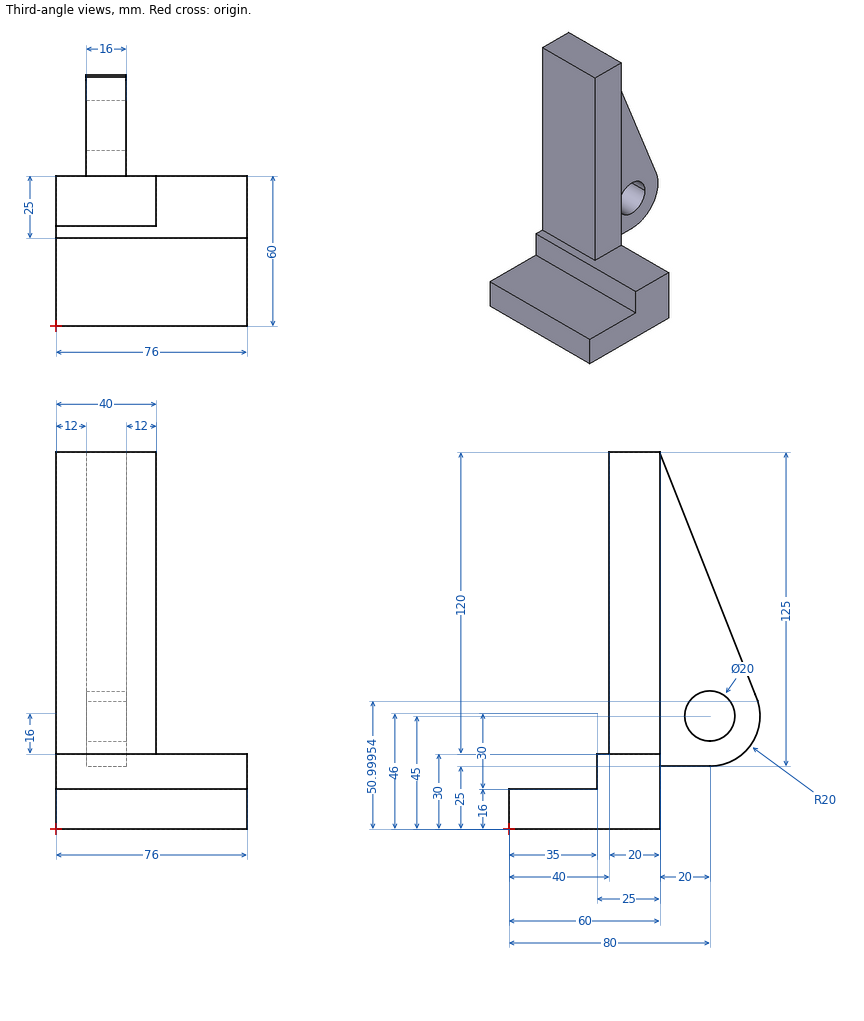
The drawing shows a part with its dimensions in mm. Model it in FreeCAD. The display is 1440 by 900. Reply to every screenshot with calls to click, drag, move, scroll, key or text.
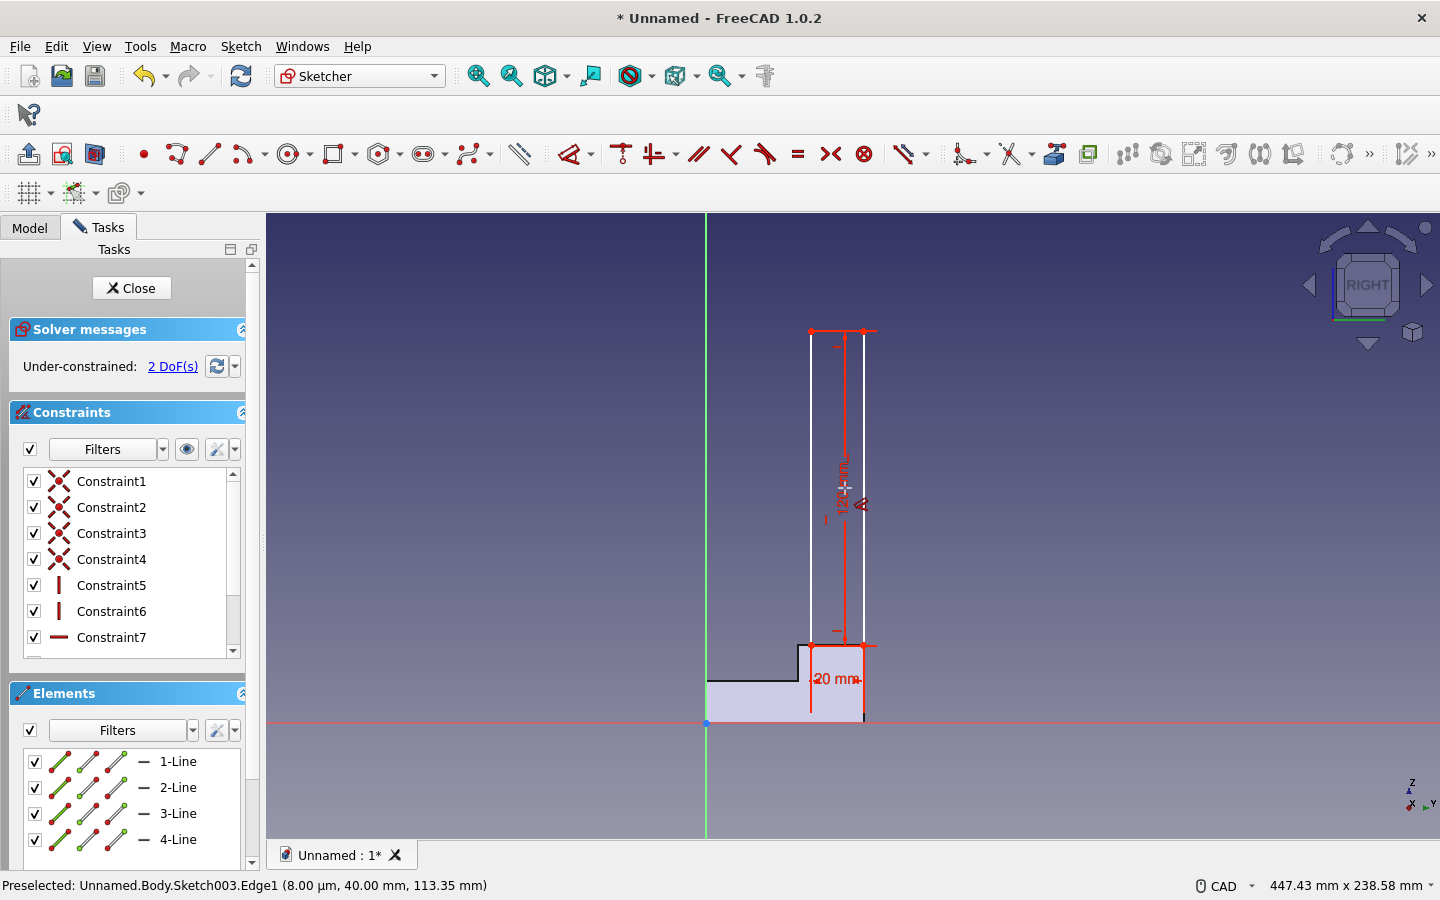
click(811, 331)
click(759, 757)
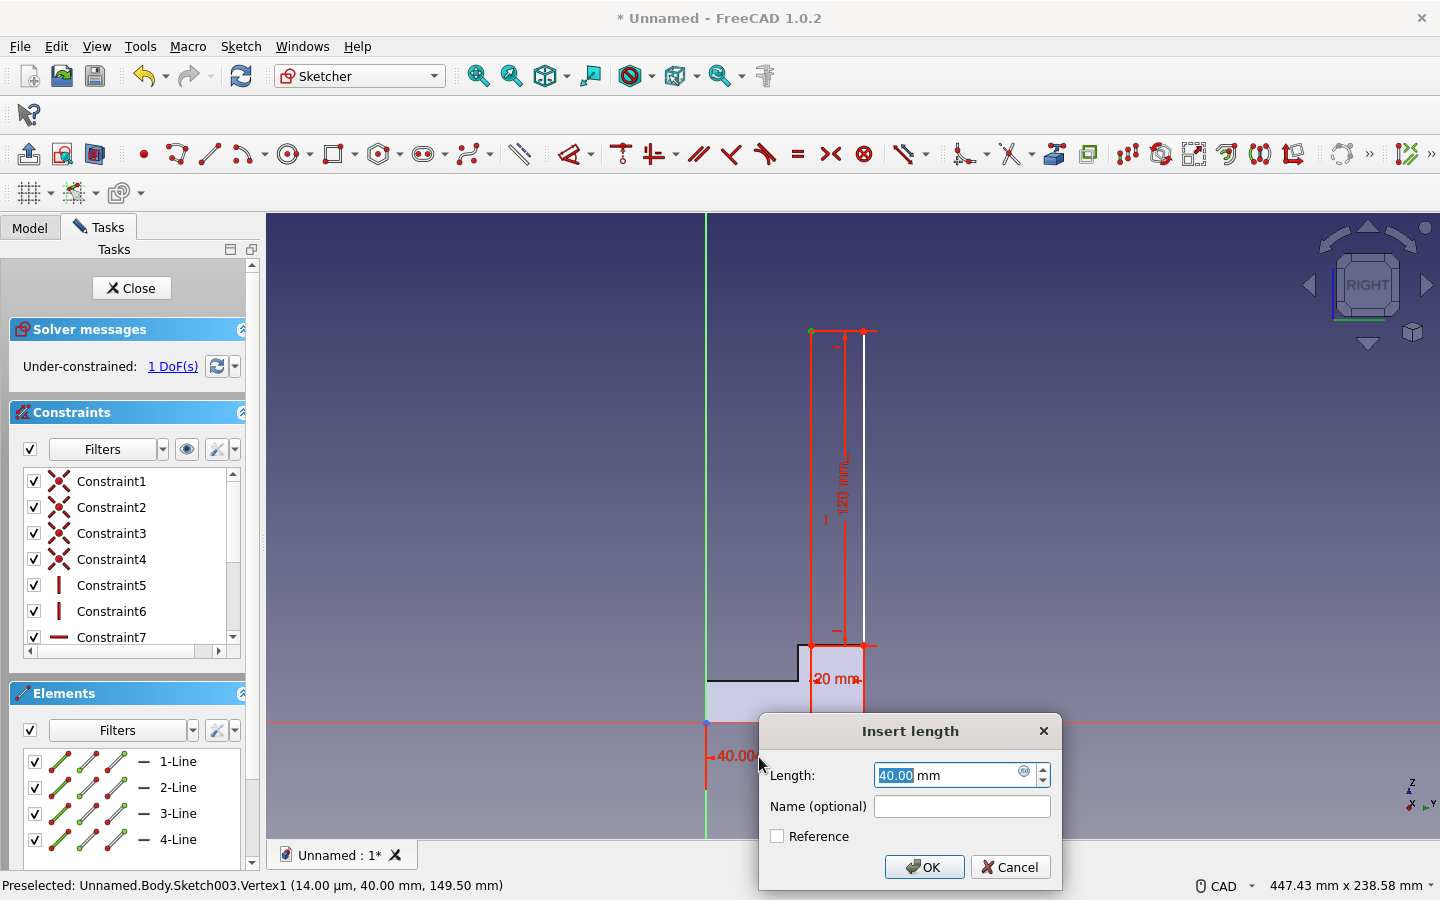
text(40)
key(Return)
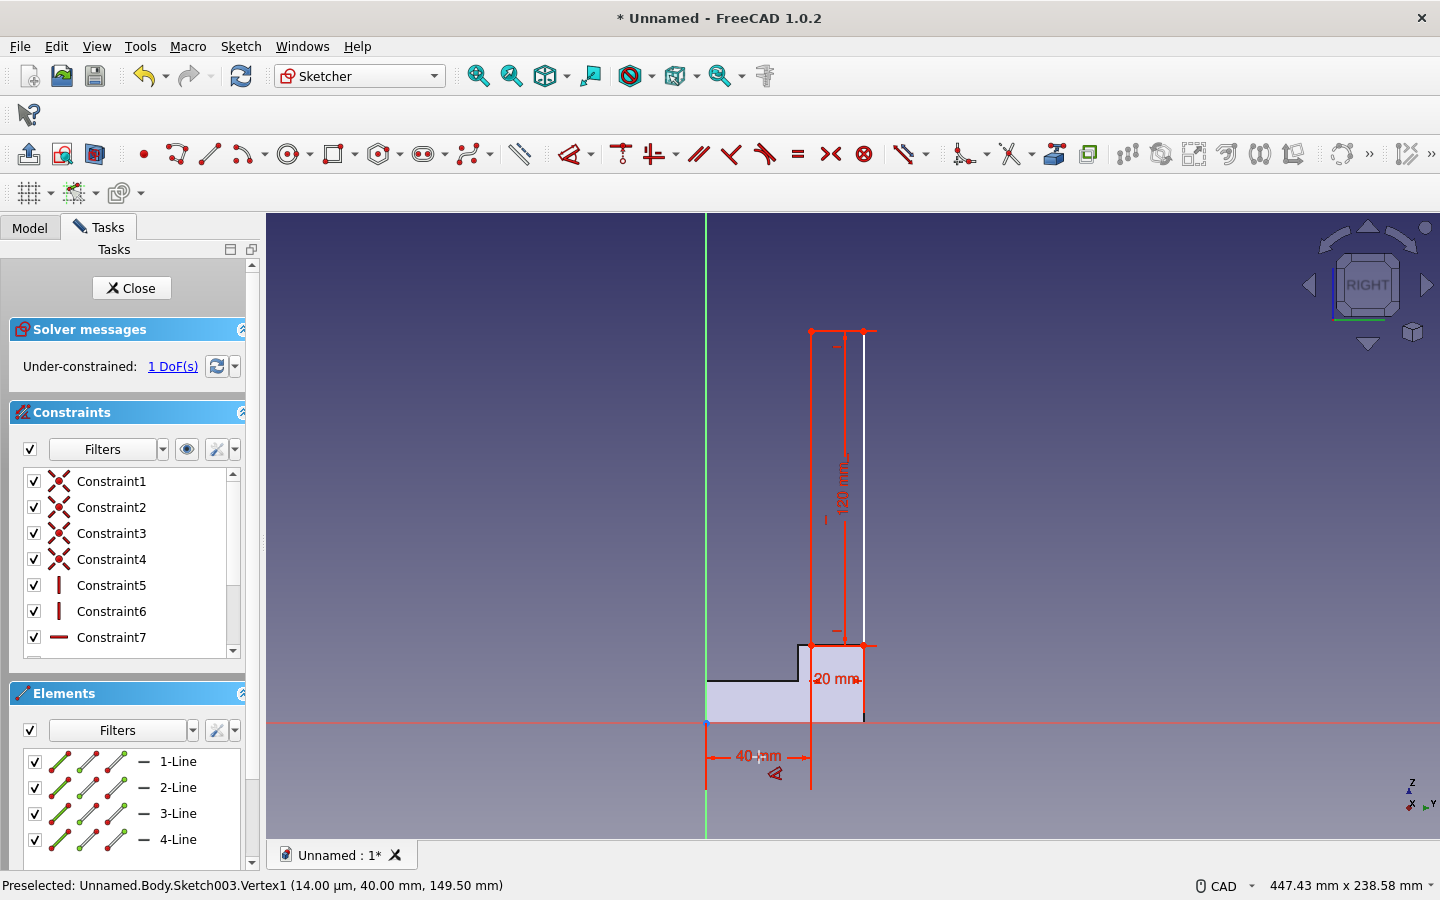
click(811, 646)
click(672, 685)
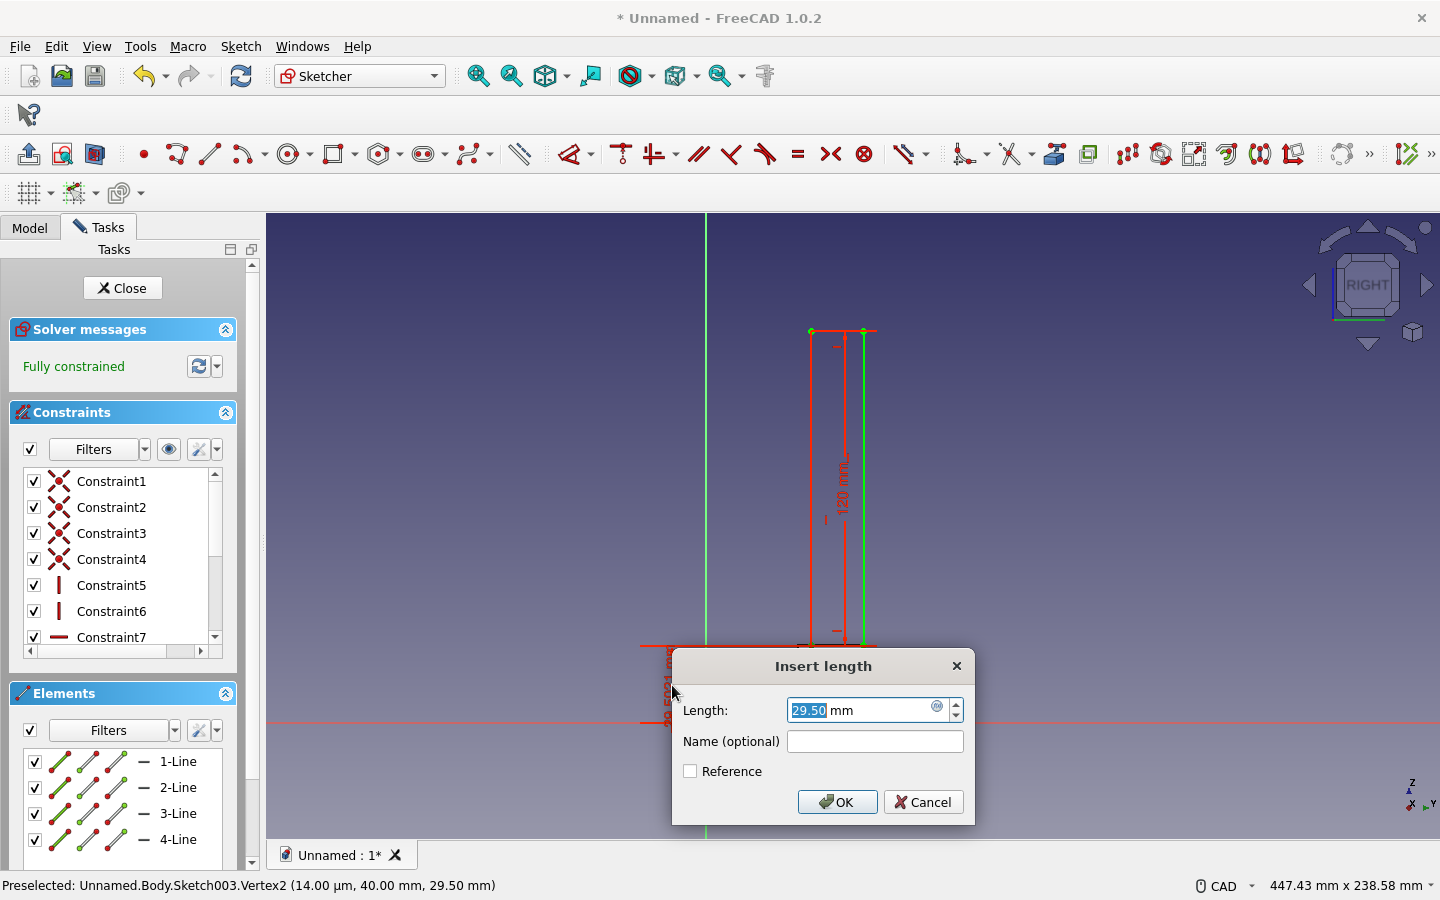
text(30)
key(Return)
key(Escape)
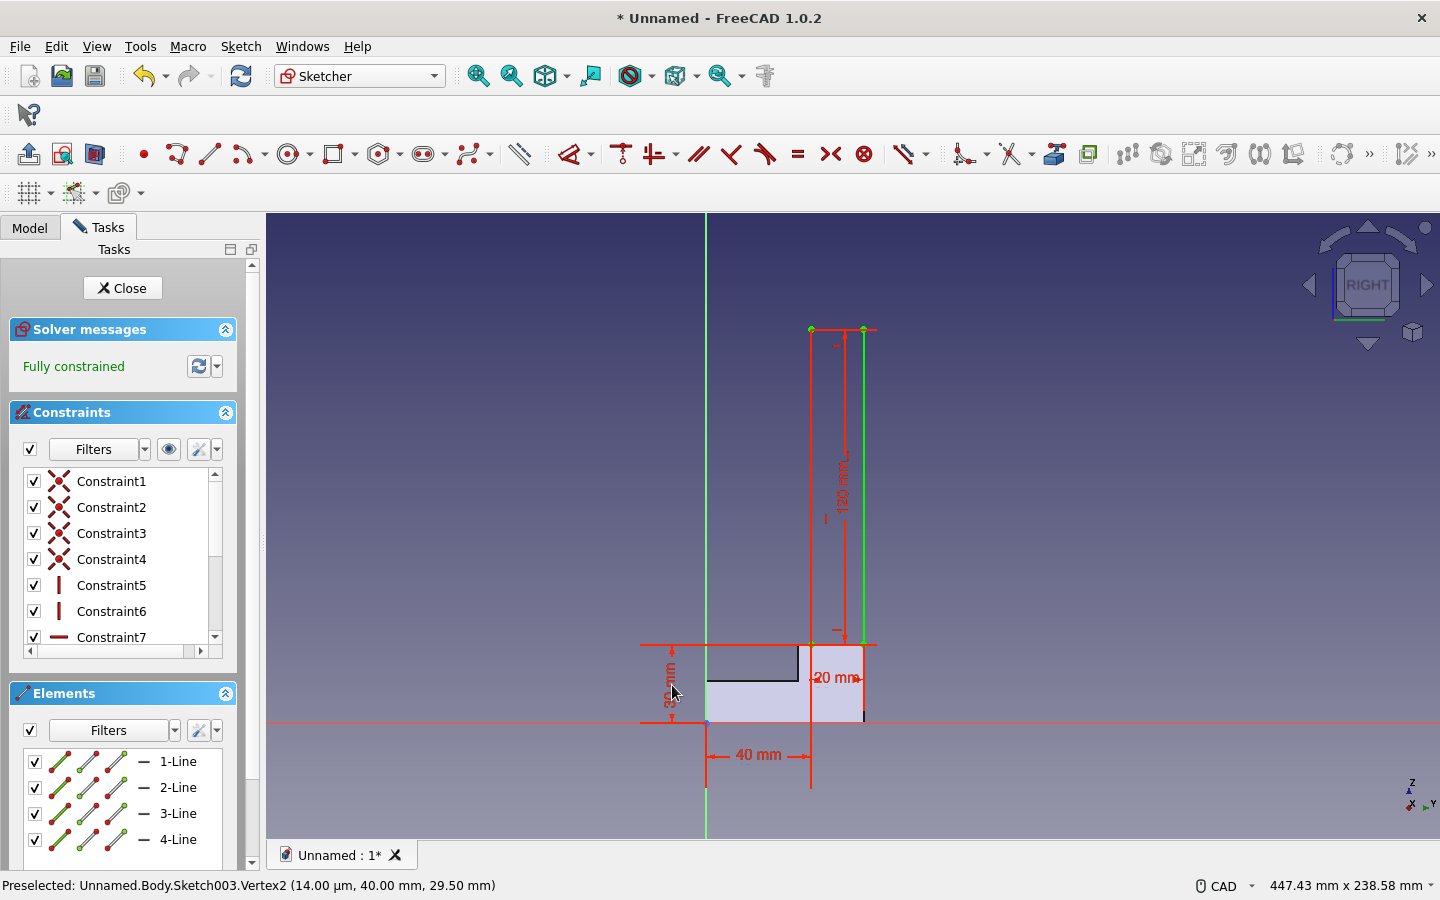
click(123, 288)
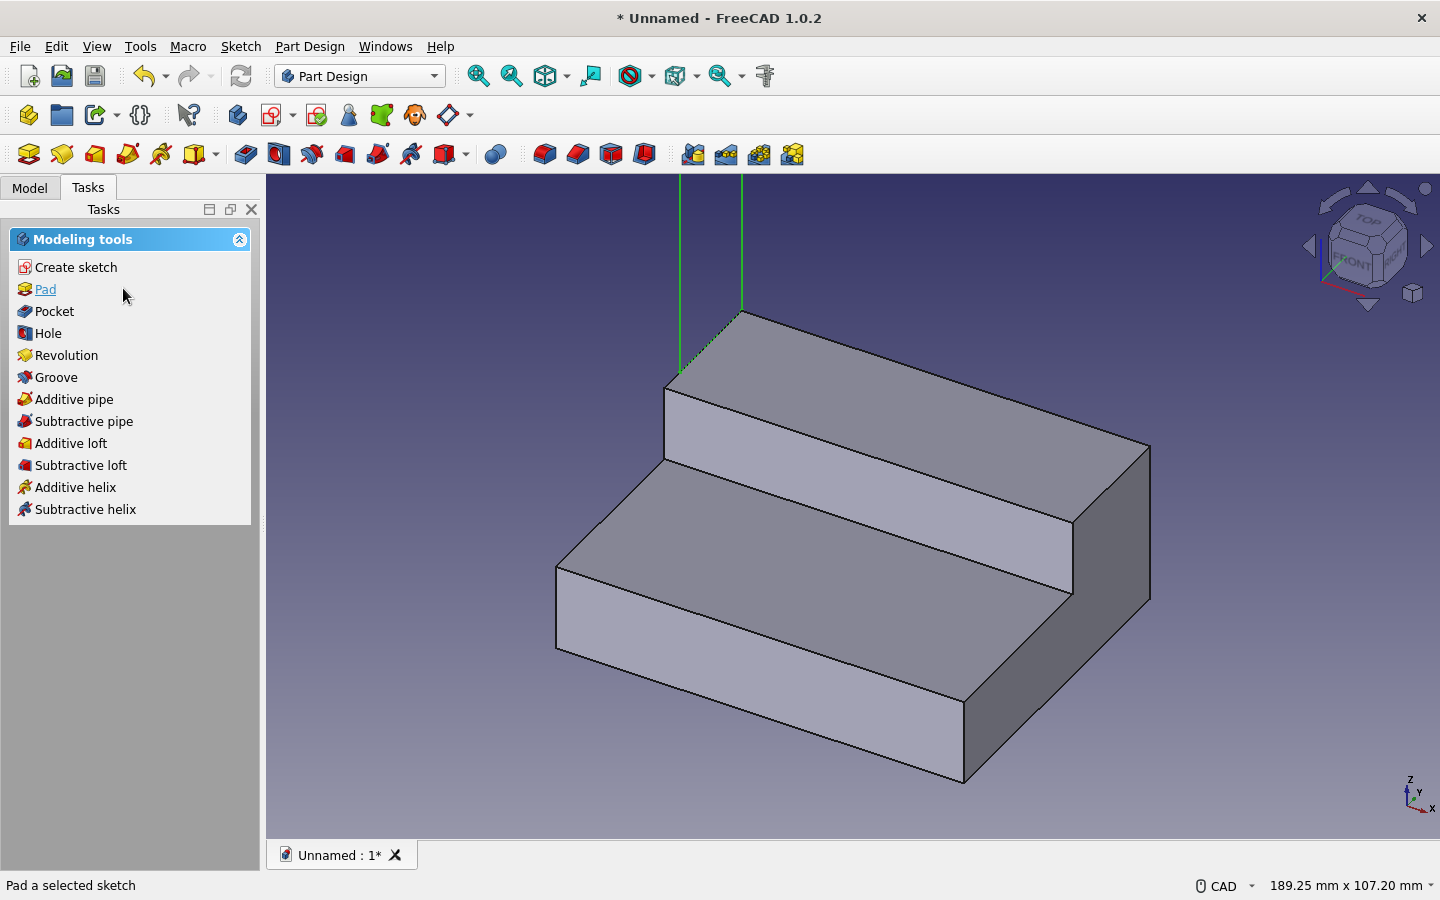
click(29, 154)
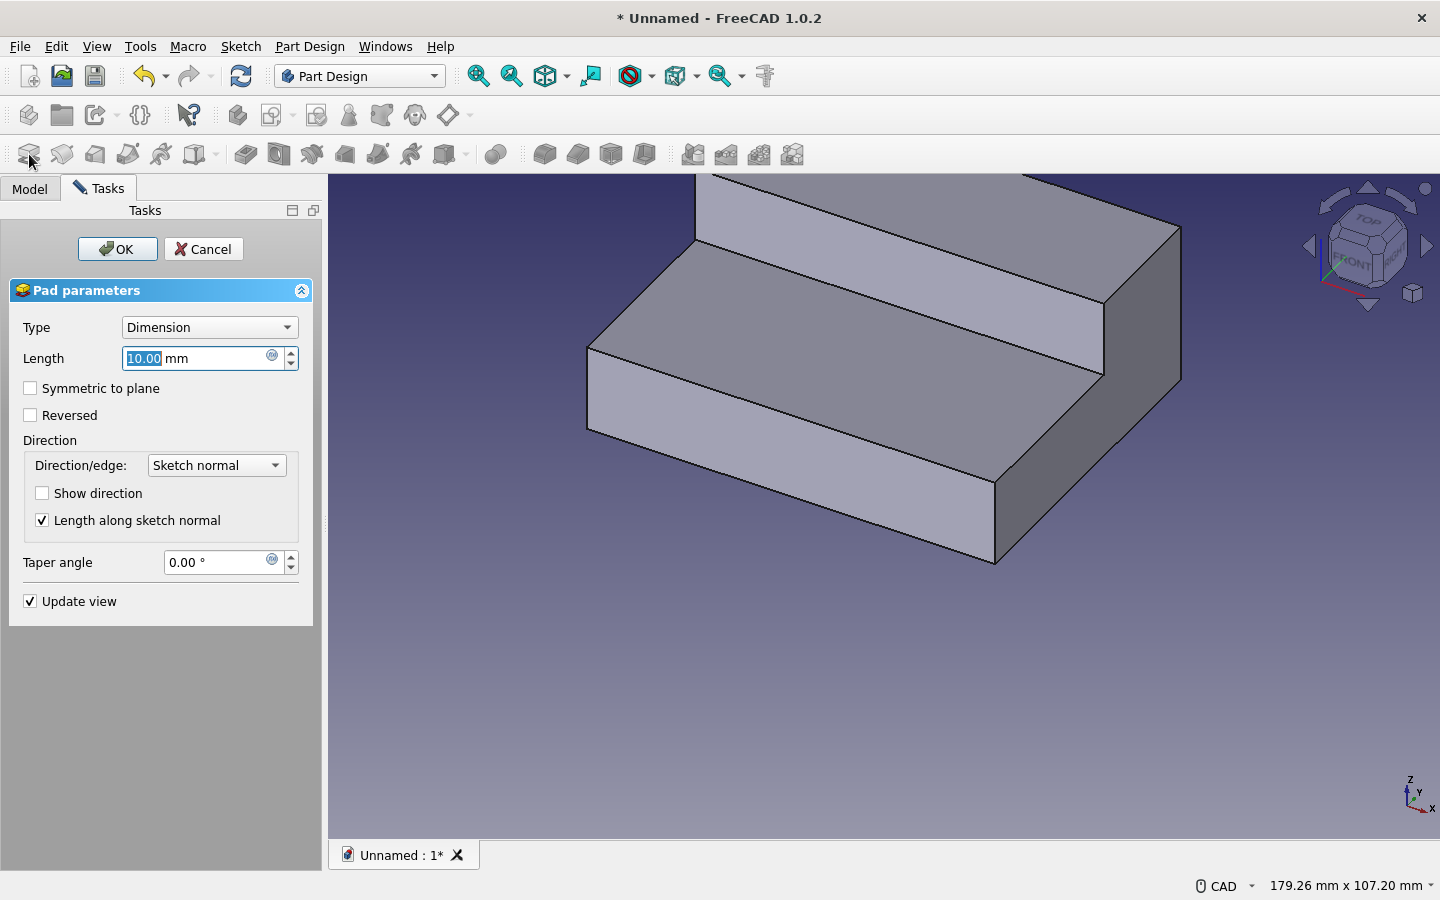
text(40)
key(Tab)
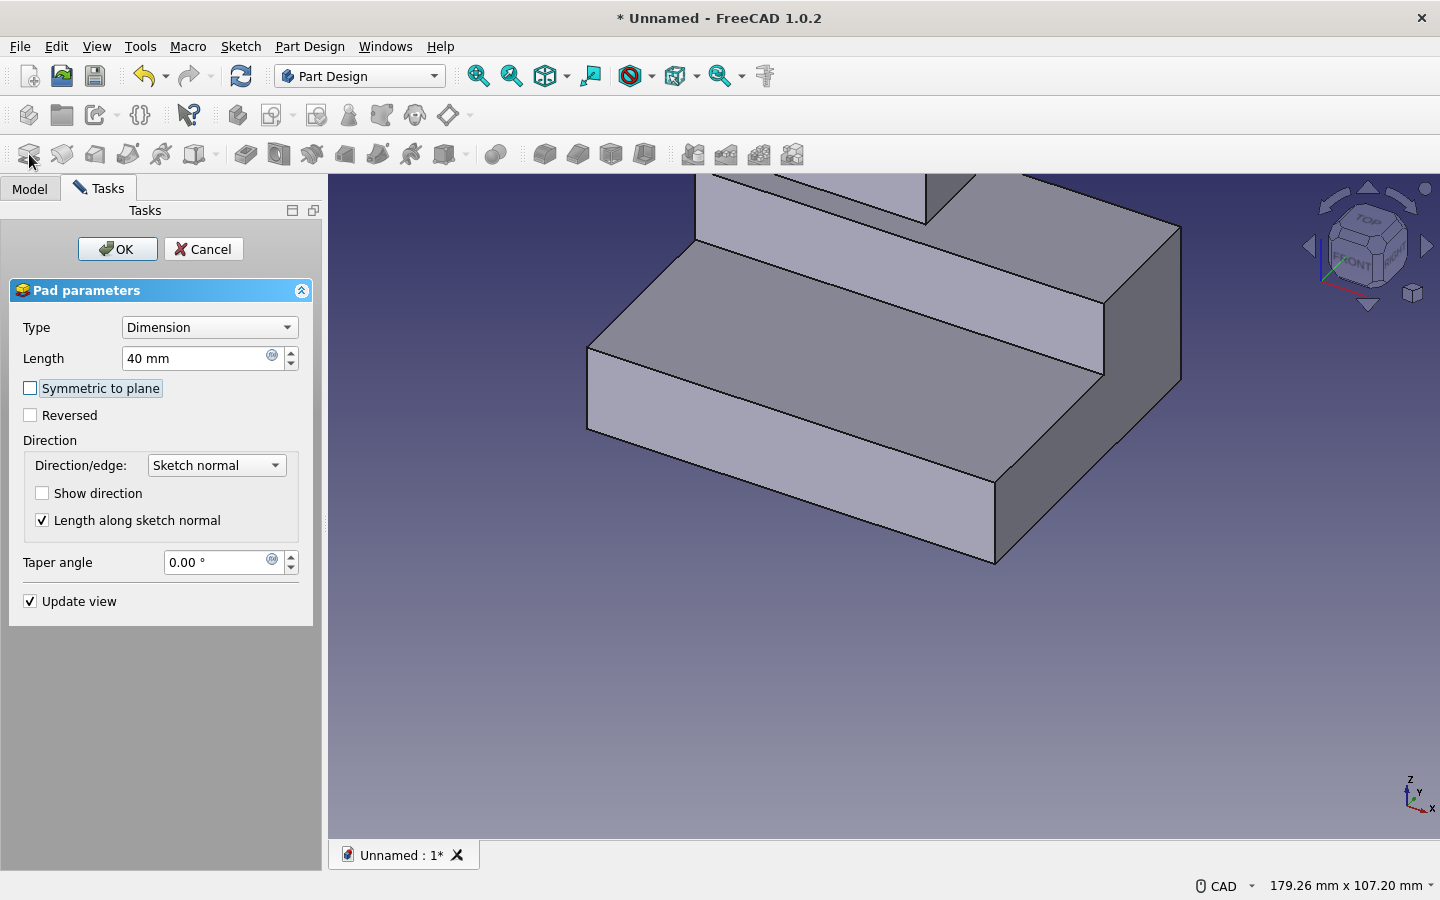
click(118, 249)